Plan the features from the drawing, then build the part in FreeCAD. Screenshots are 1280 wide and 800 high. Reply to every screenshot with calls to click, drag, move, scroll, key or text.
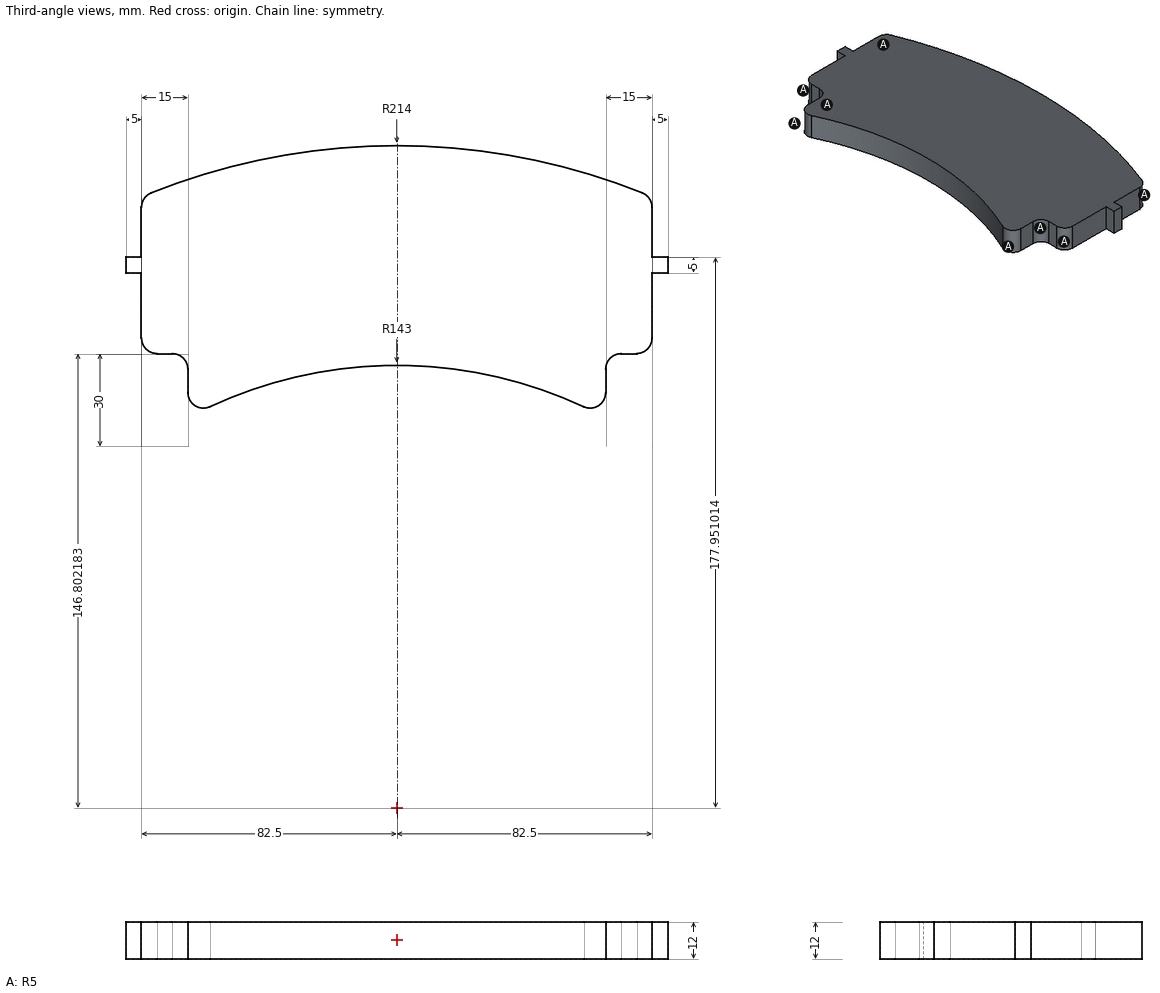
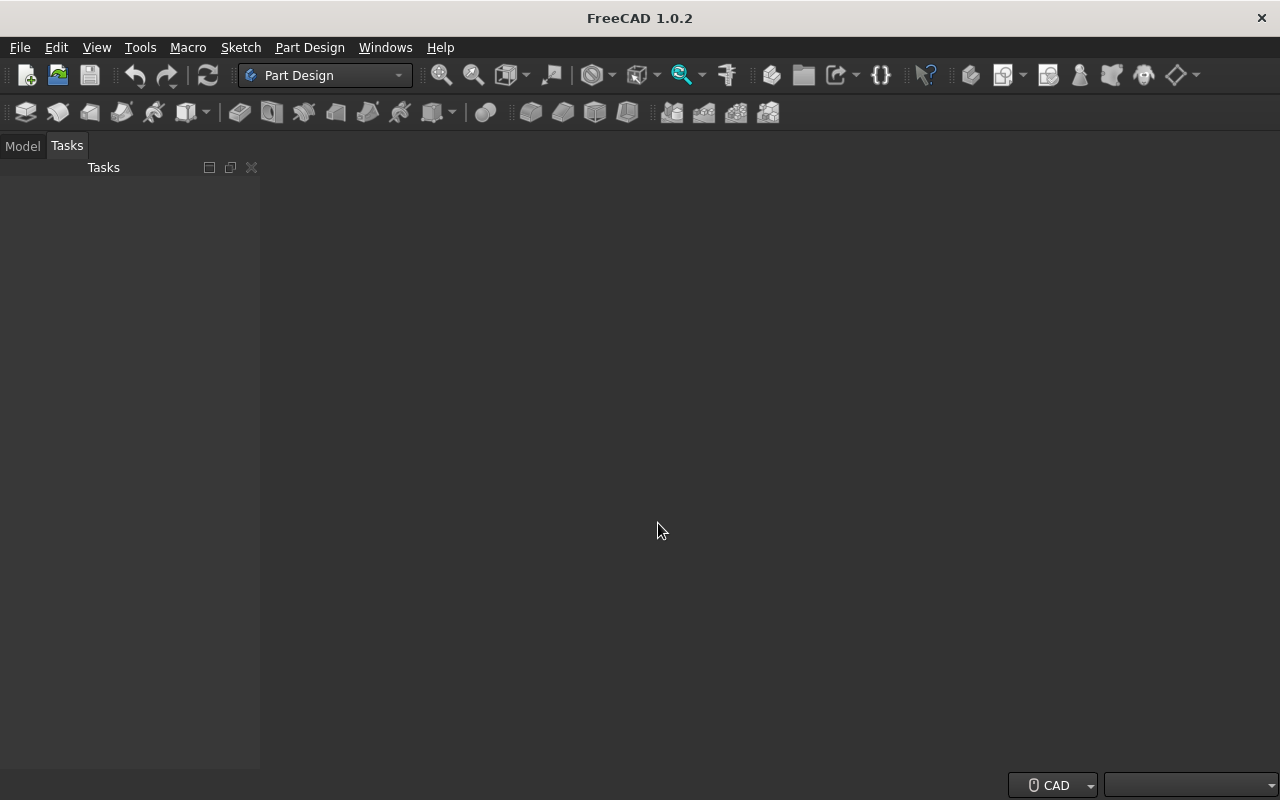
click(26, 76)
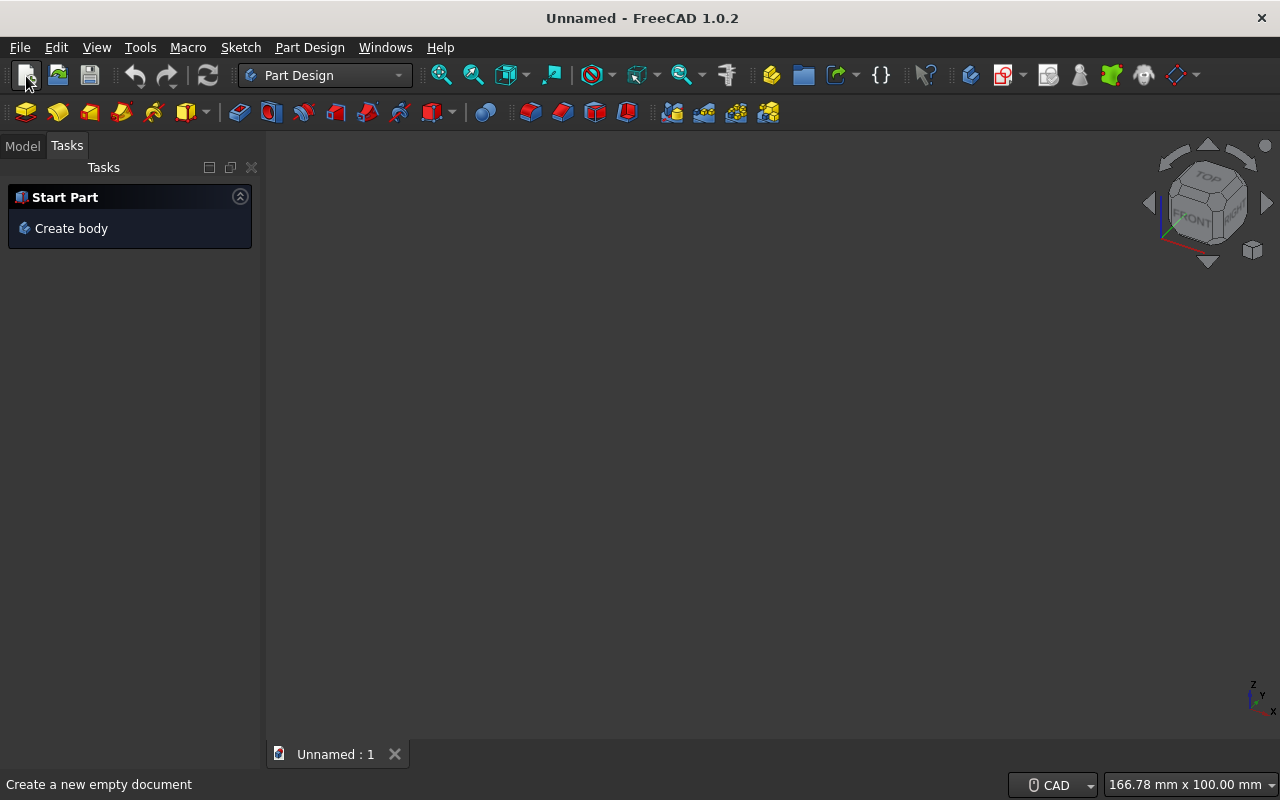
click(1004, 76)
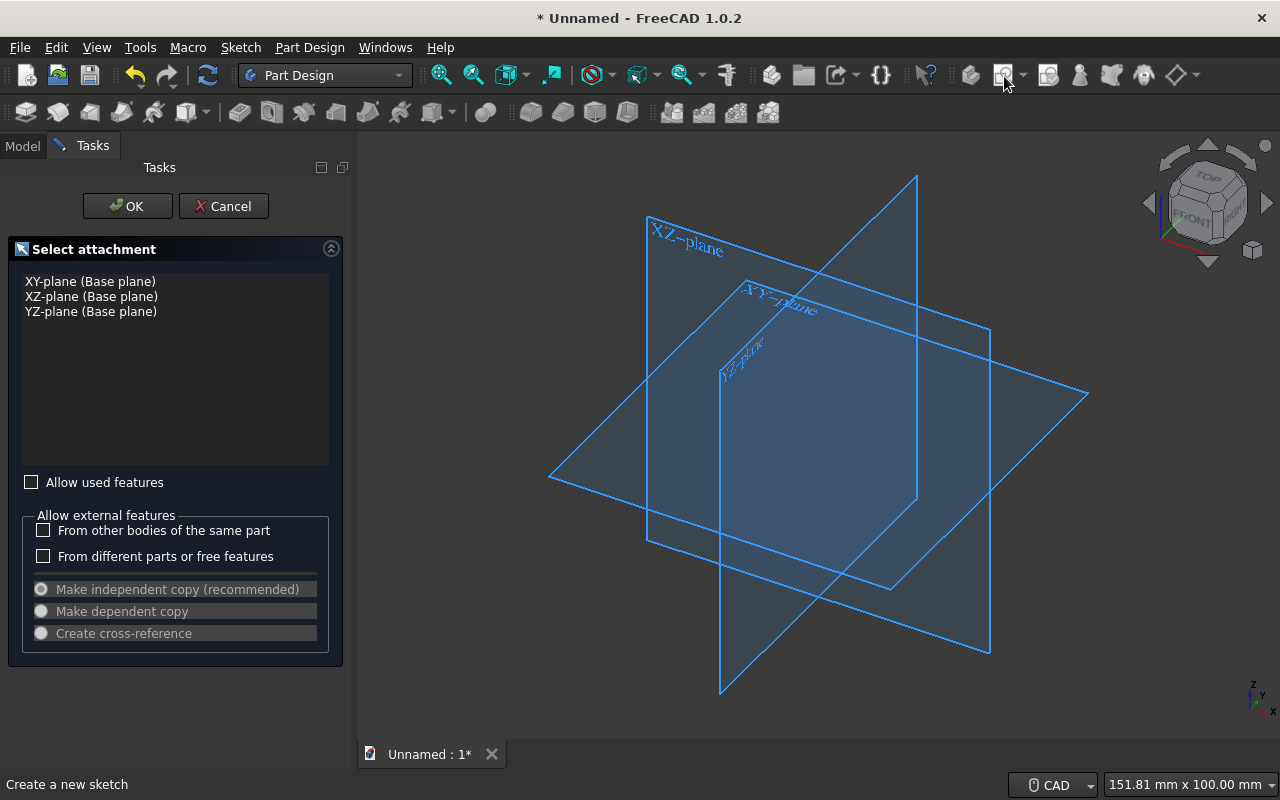
click(82, 282)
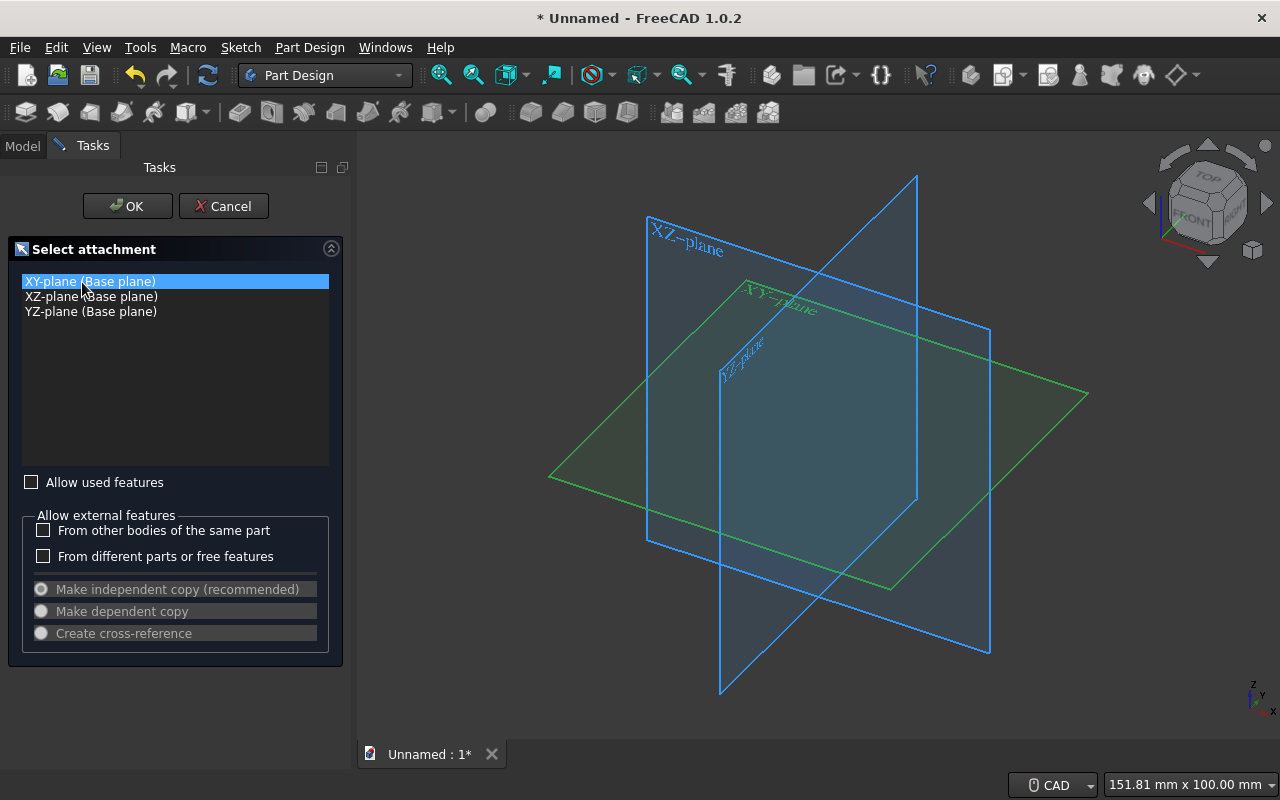
click(128, 206)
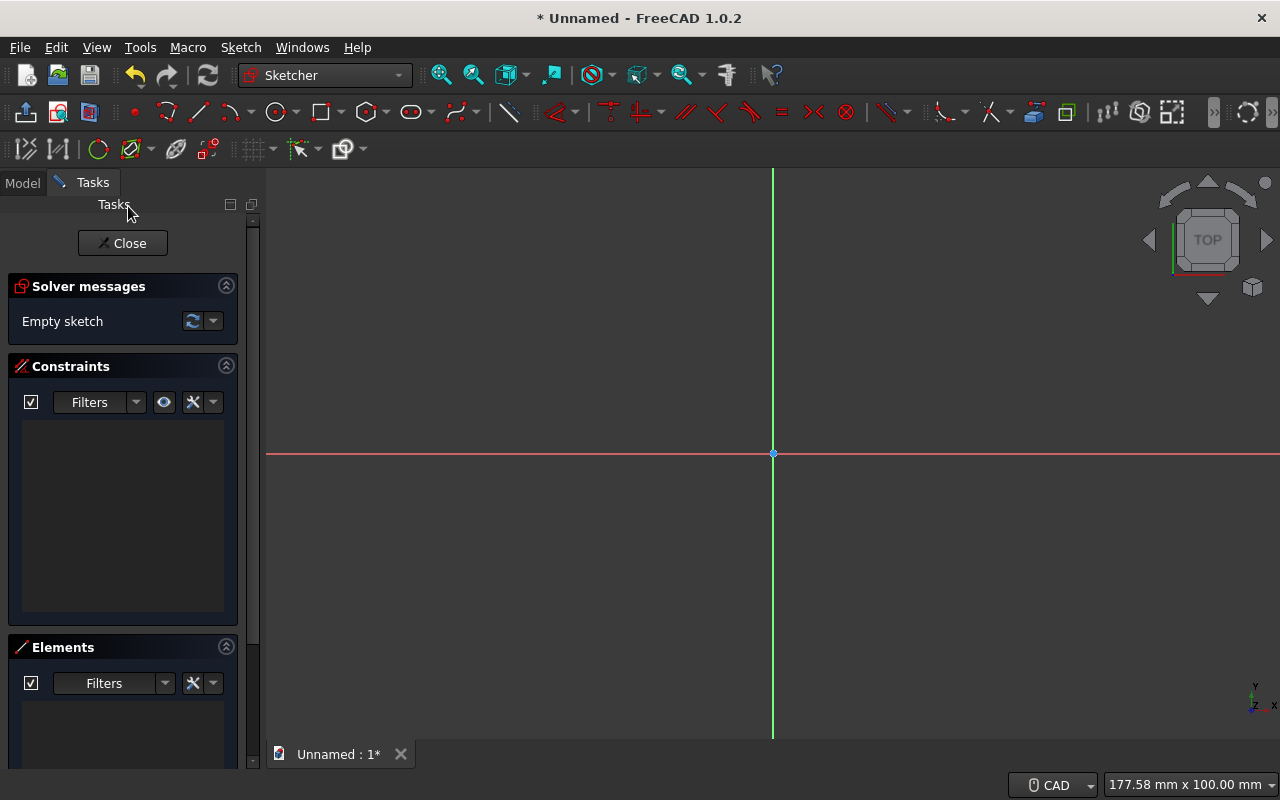
scroll(675, 711, down, 6)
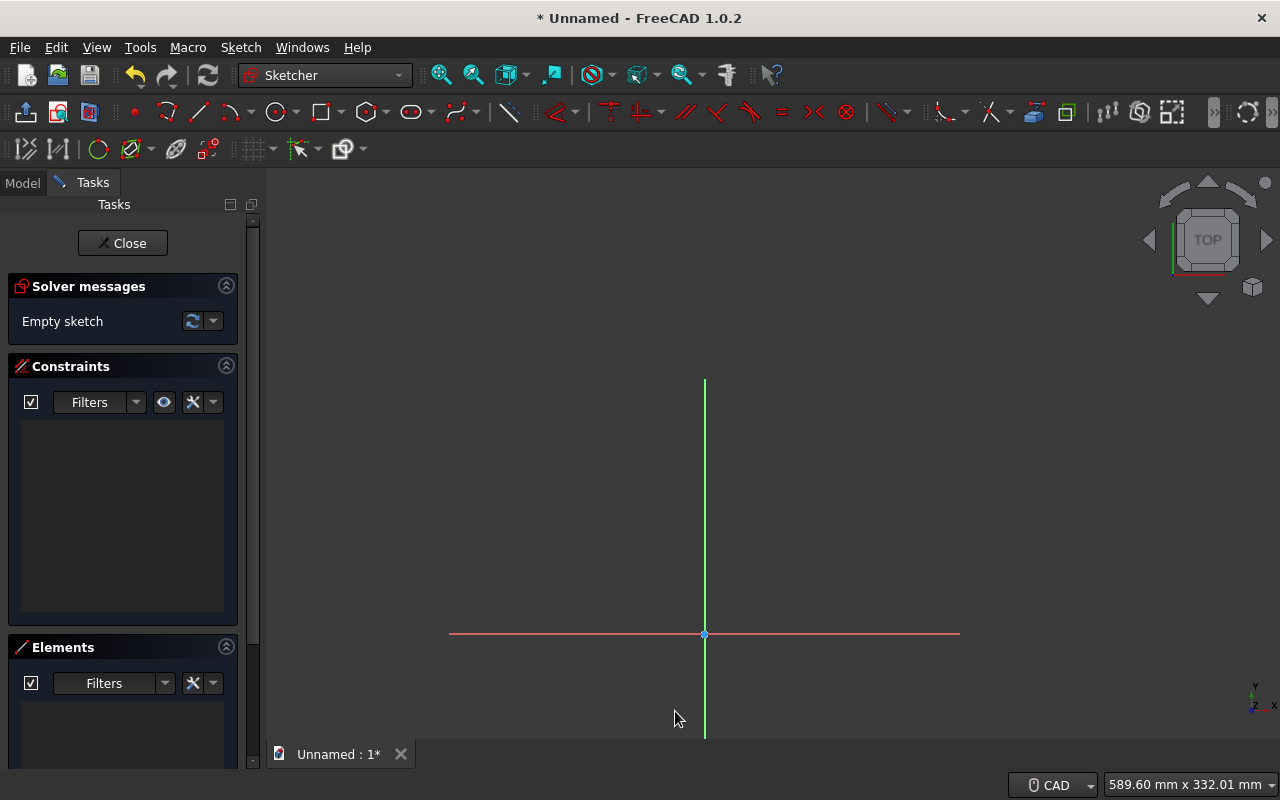
click(200, 112)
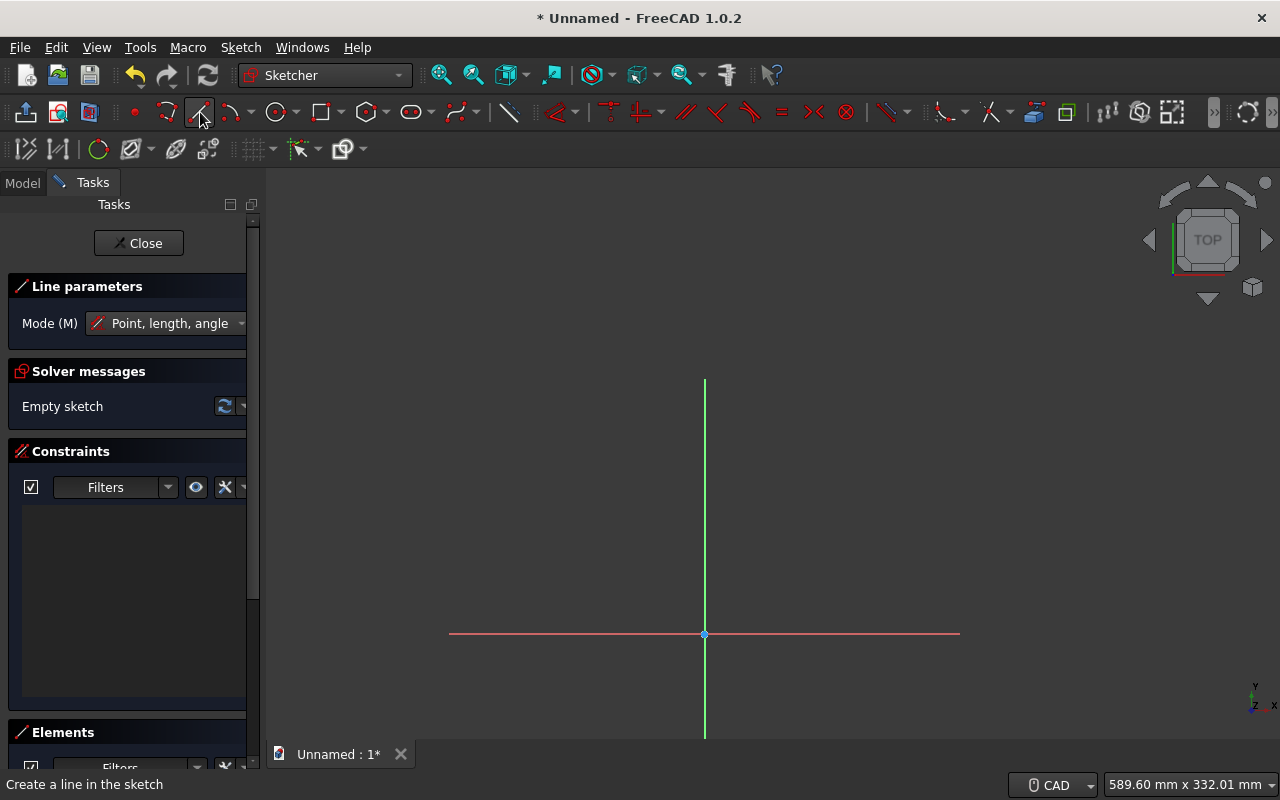
click(563, 295)
click(563, 433)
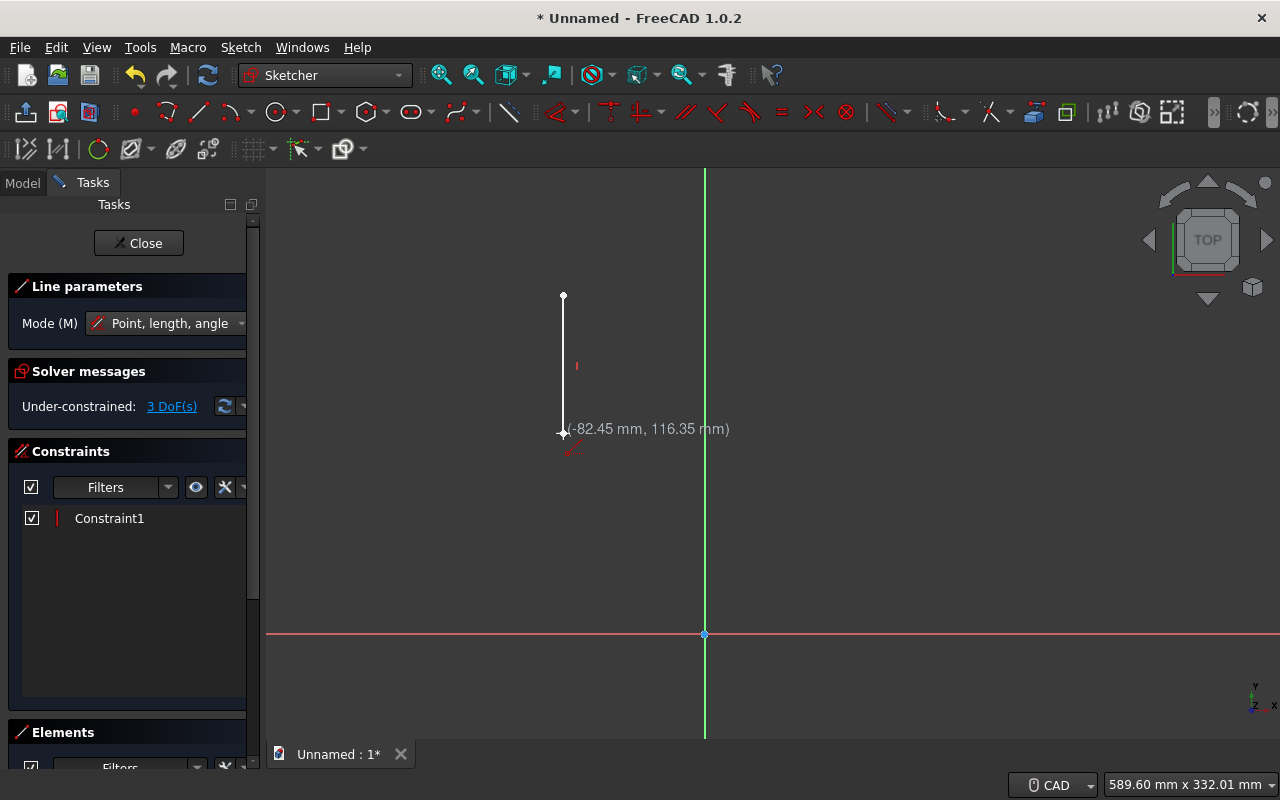
click(847, 433)
click(847, 295)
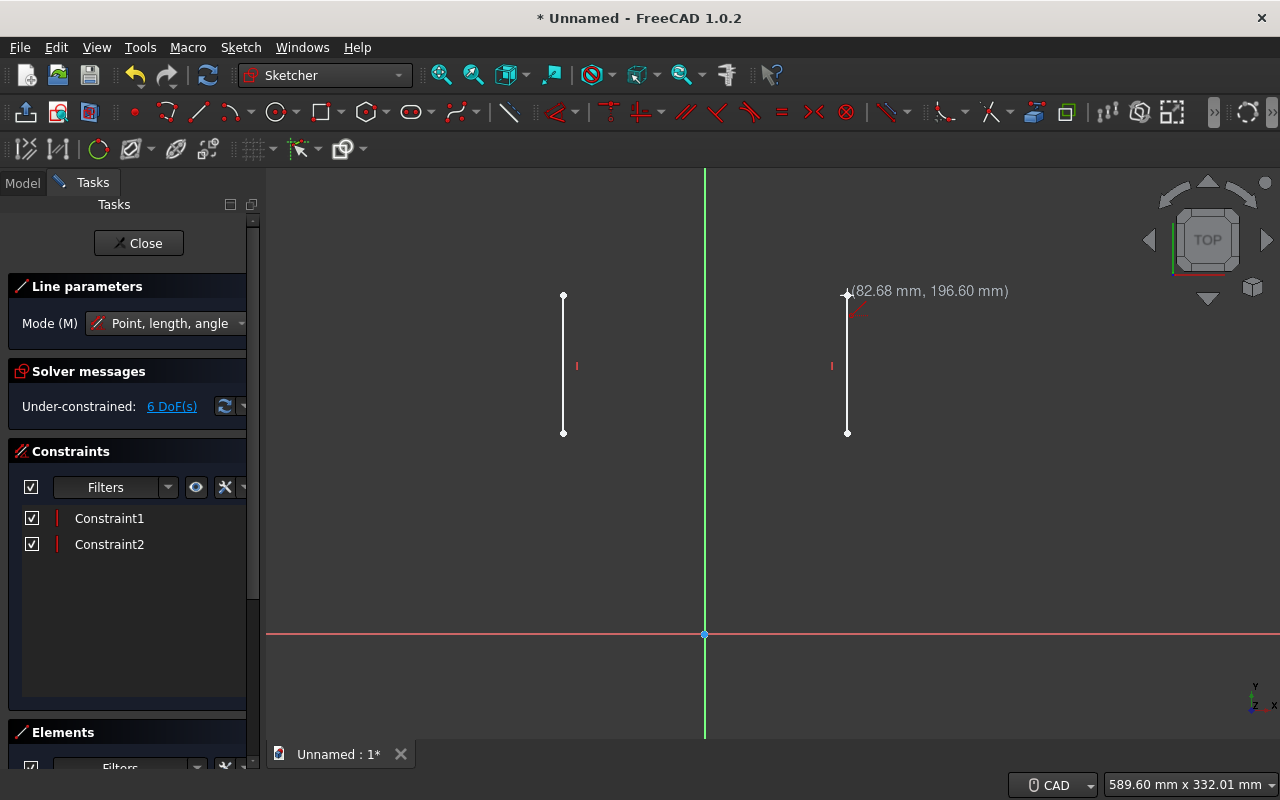
key(g)
key(3)
key(a)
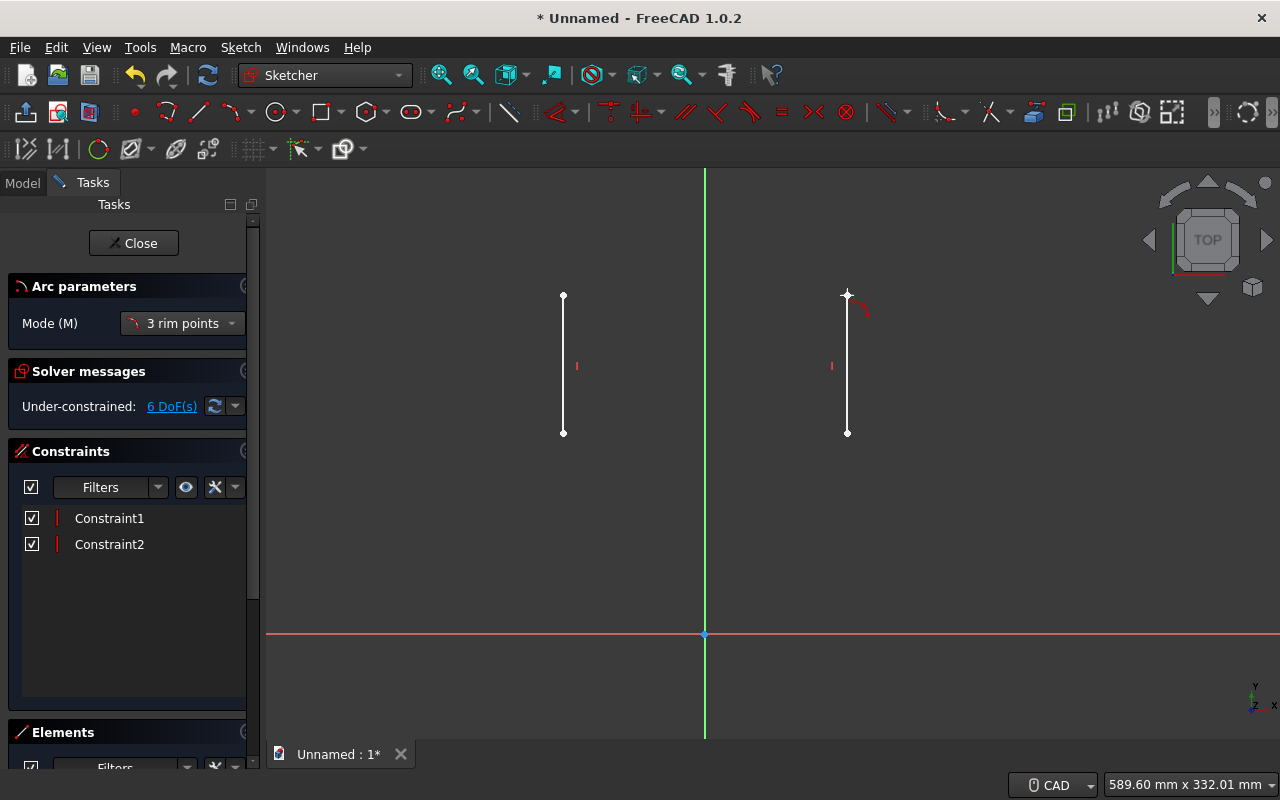
click(563, 434)
click(847, 434)
click(735, 390)